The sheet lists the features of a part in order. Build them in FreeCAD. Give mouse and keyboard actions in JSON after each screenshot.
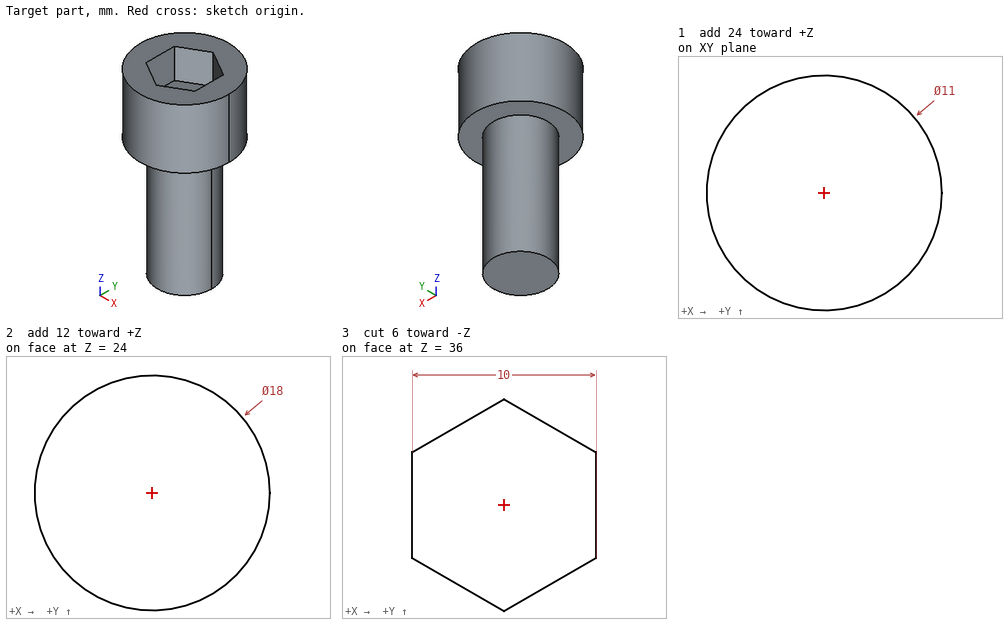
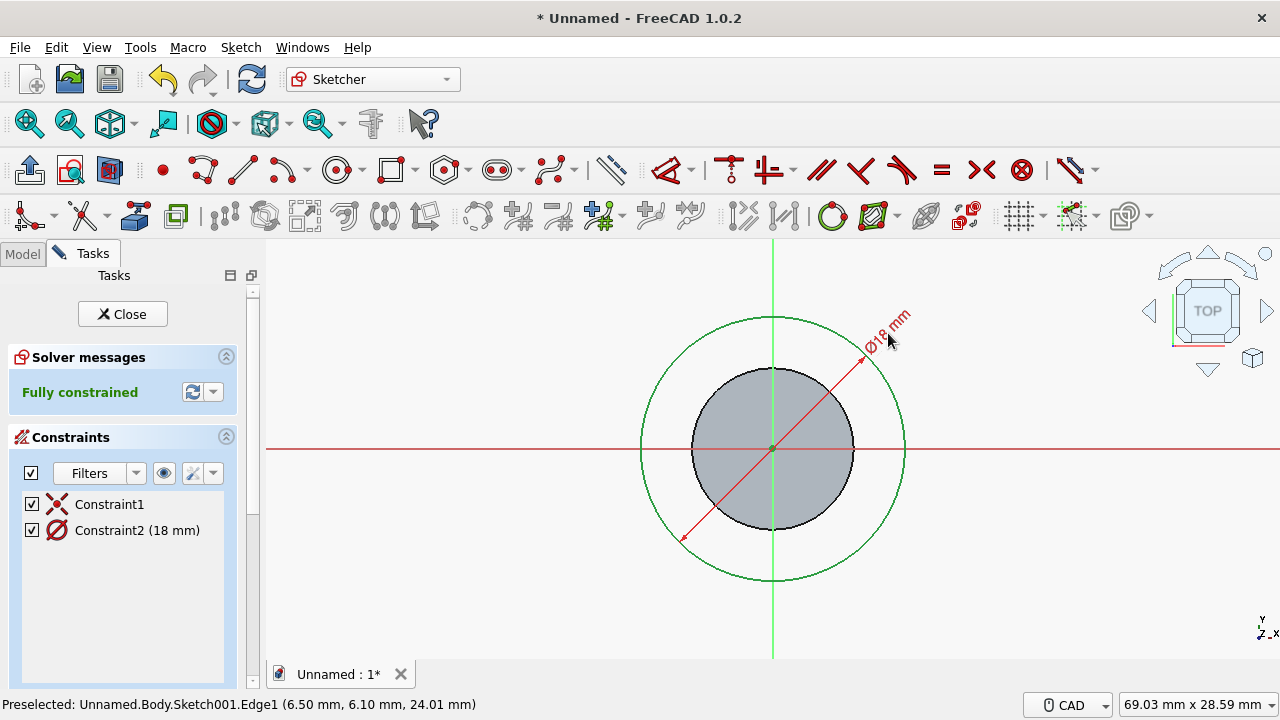
{"action": "left_click", "coordinate": [123, 314]}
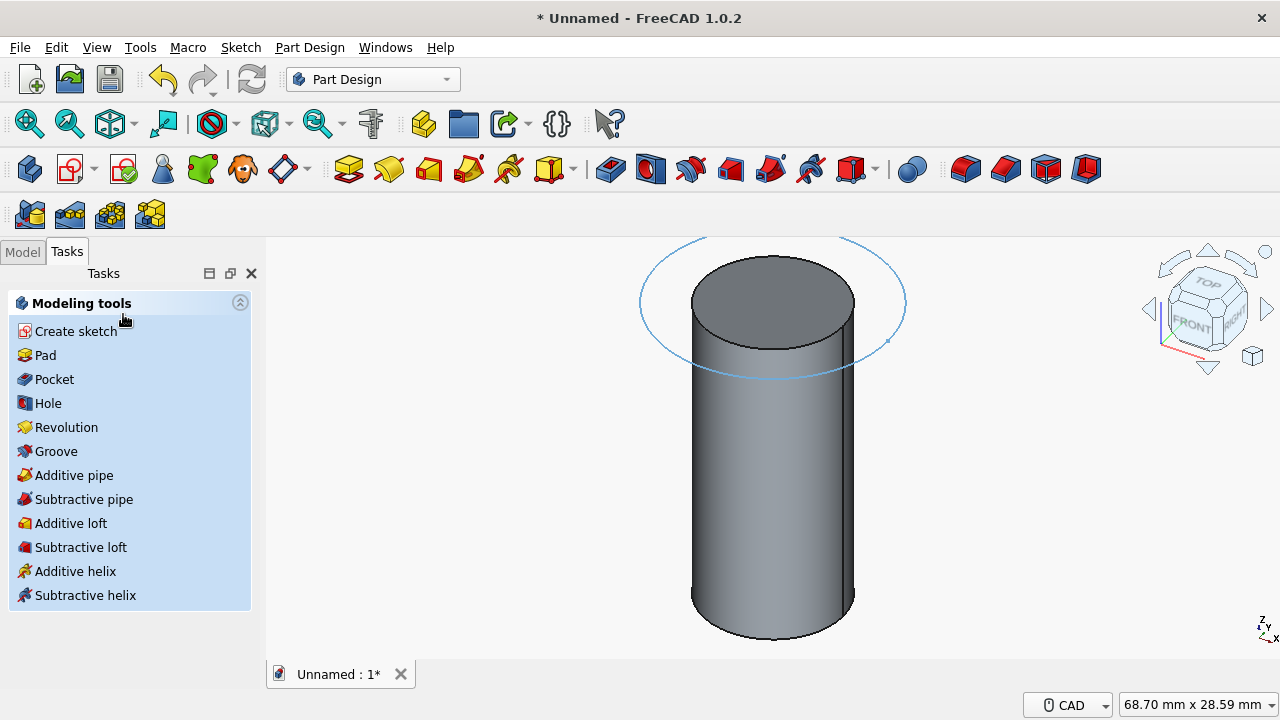
{"action": "left_click", "coordinate": [350, 170]}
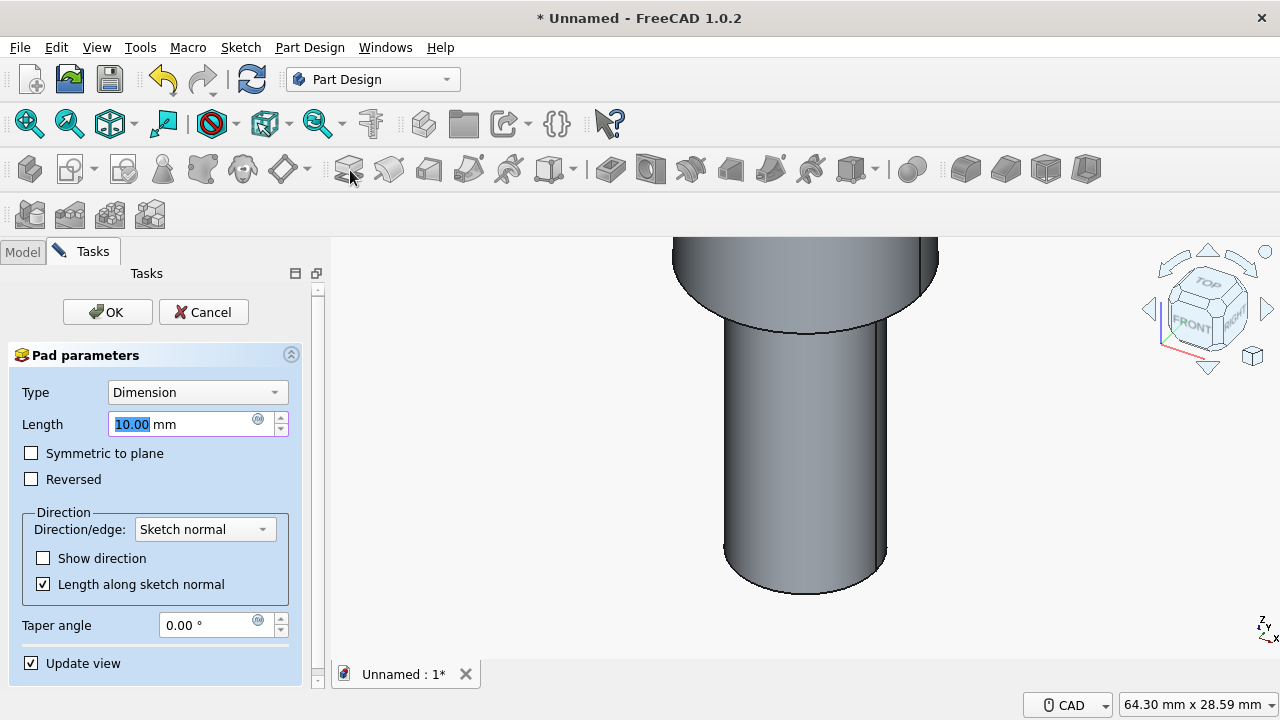
{"action": "type", "text": "12"}
{"action": "key", "text": "Tab"}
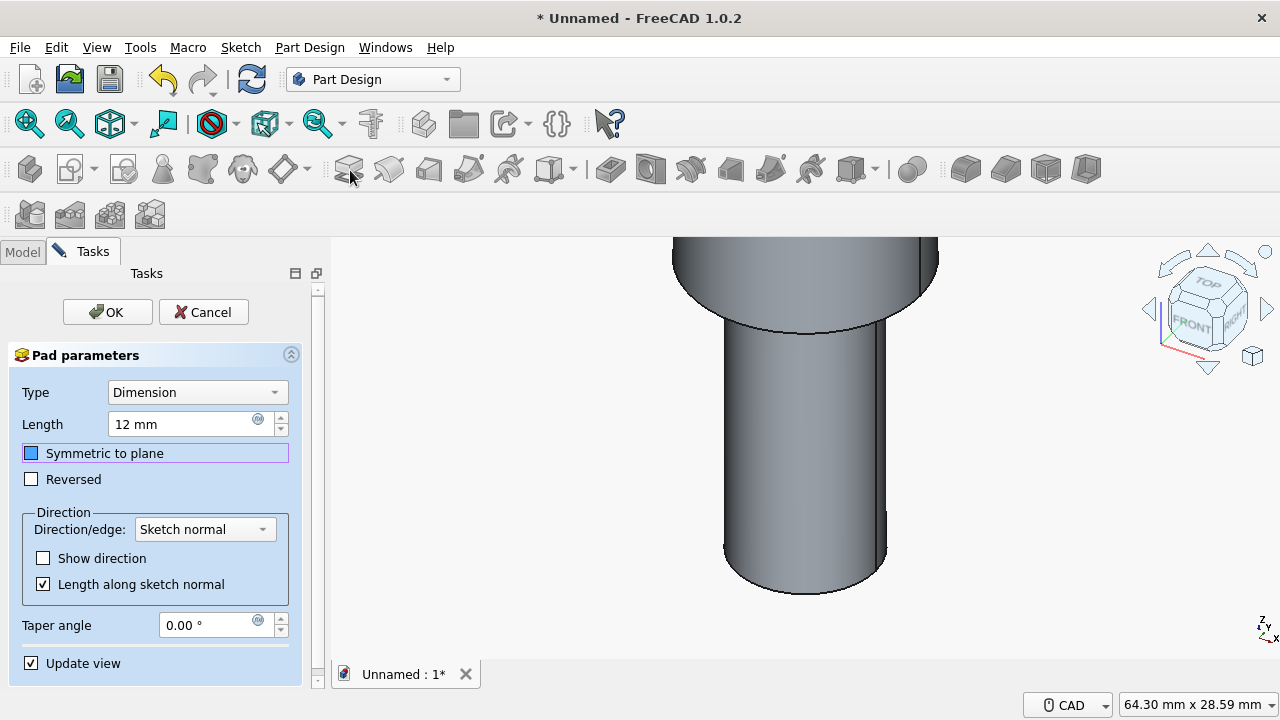
{"action": "left_click", "coordinate": [108, 312]}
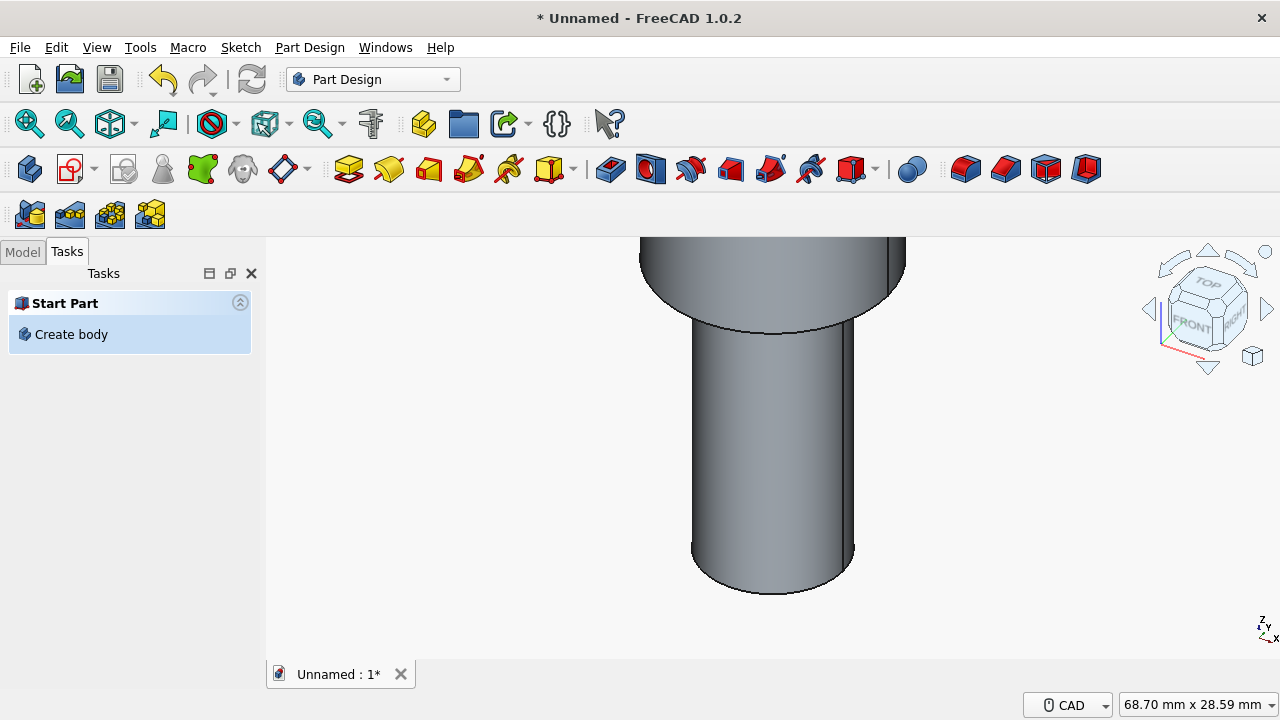
{"action": "left_click", "coordinate": [30, 124]}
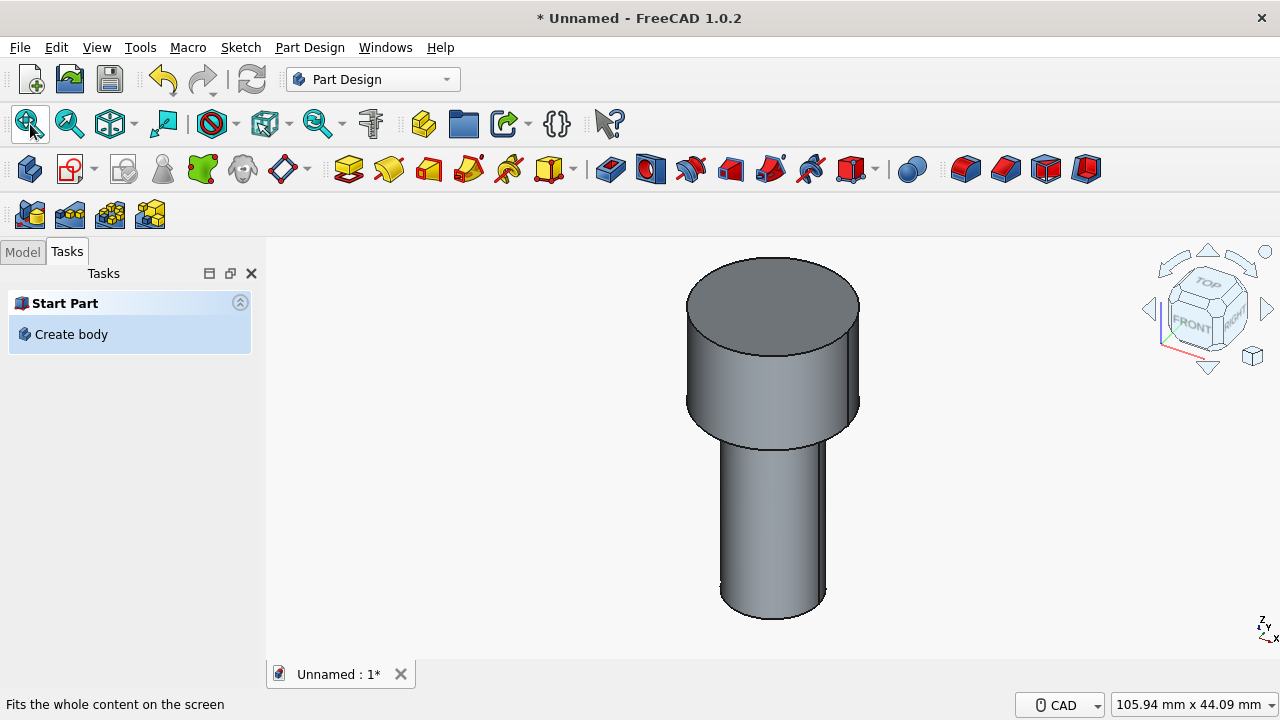
{"action": "left_click", "coordinate": [773, 306]}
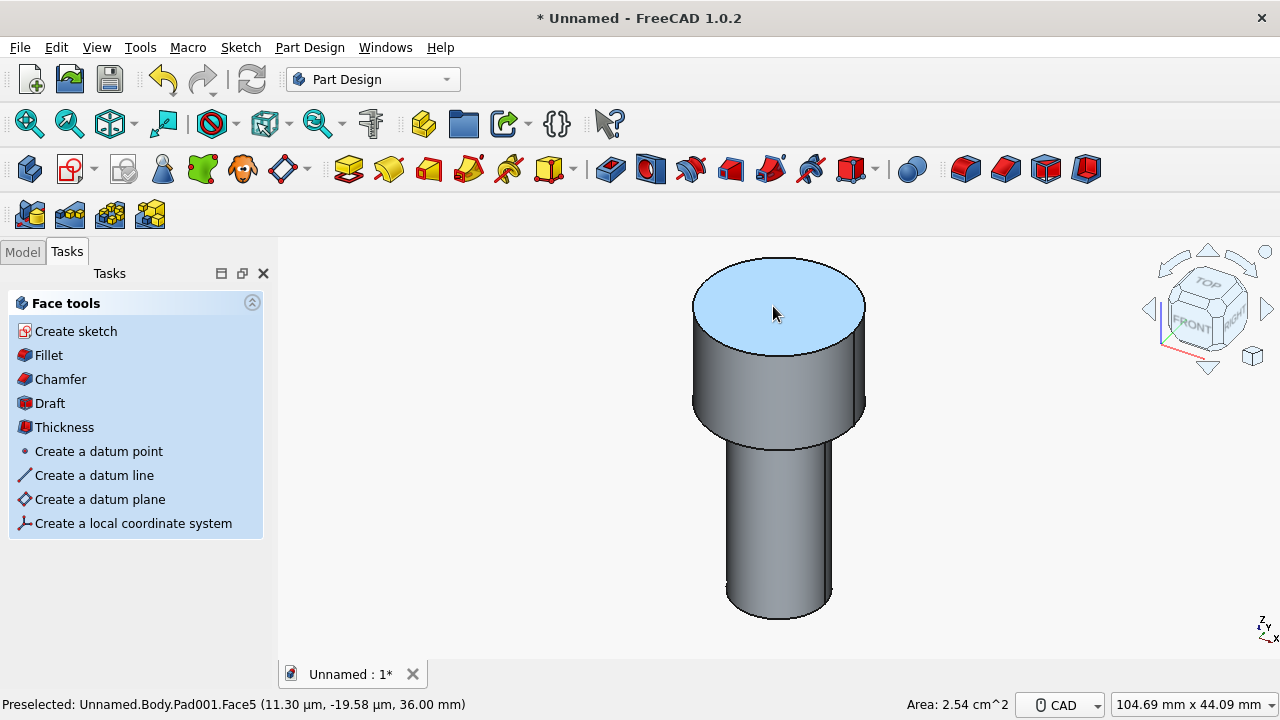
{"action": "left_click", "coordinate": [70, 170]}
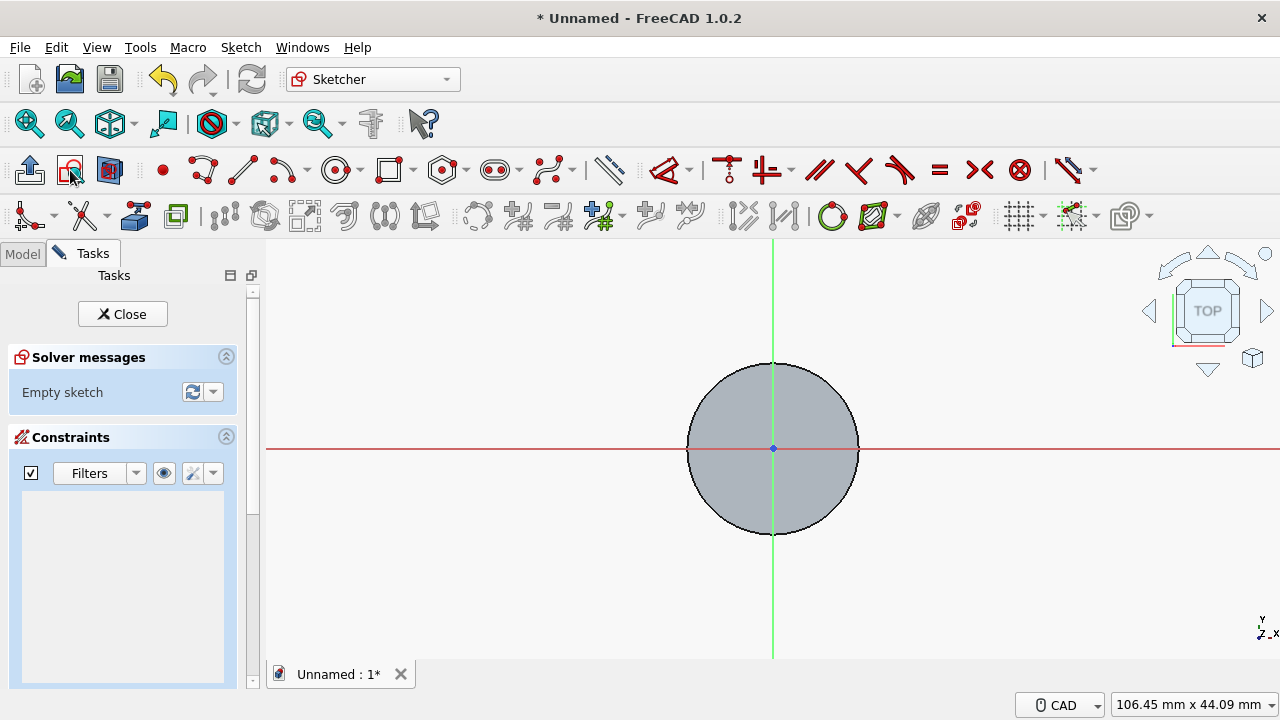
{"action": "scroll", "coordinate": [829, 449], "scroll_direction": "up", "scroll_amount": 4}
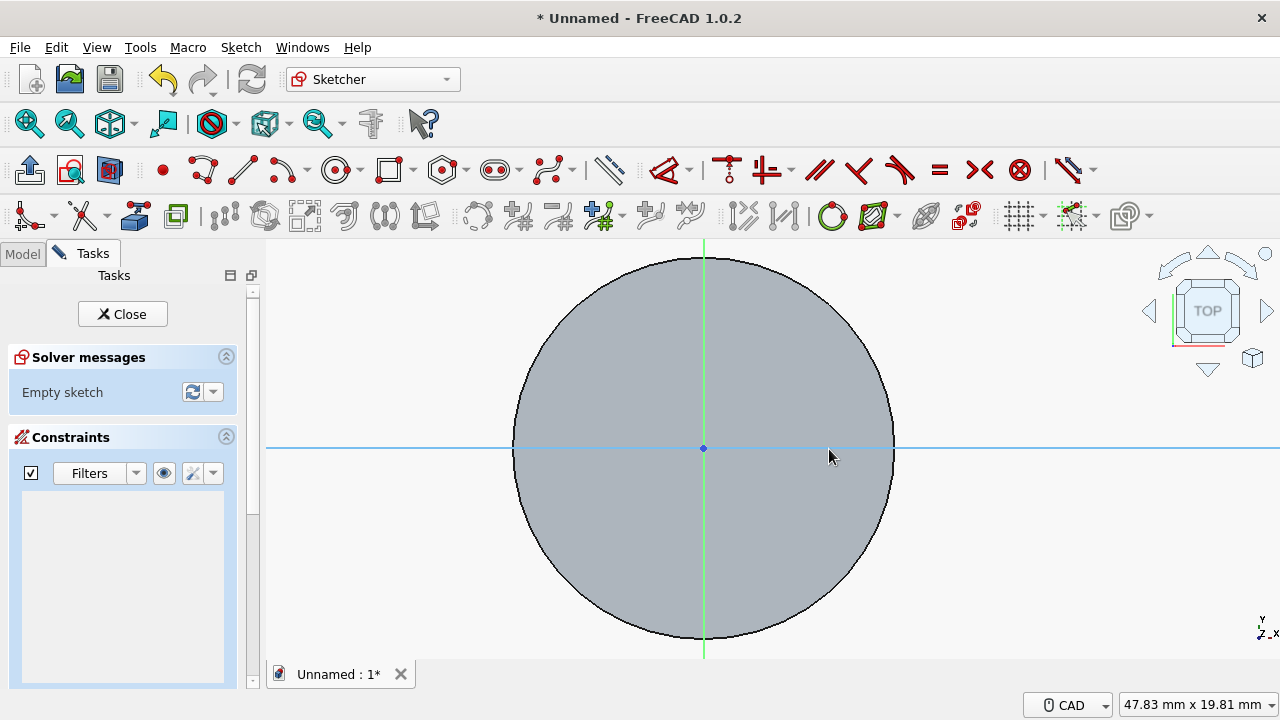
{"action": "left_click", "coordinate": [442, 170]}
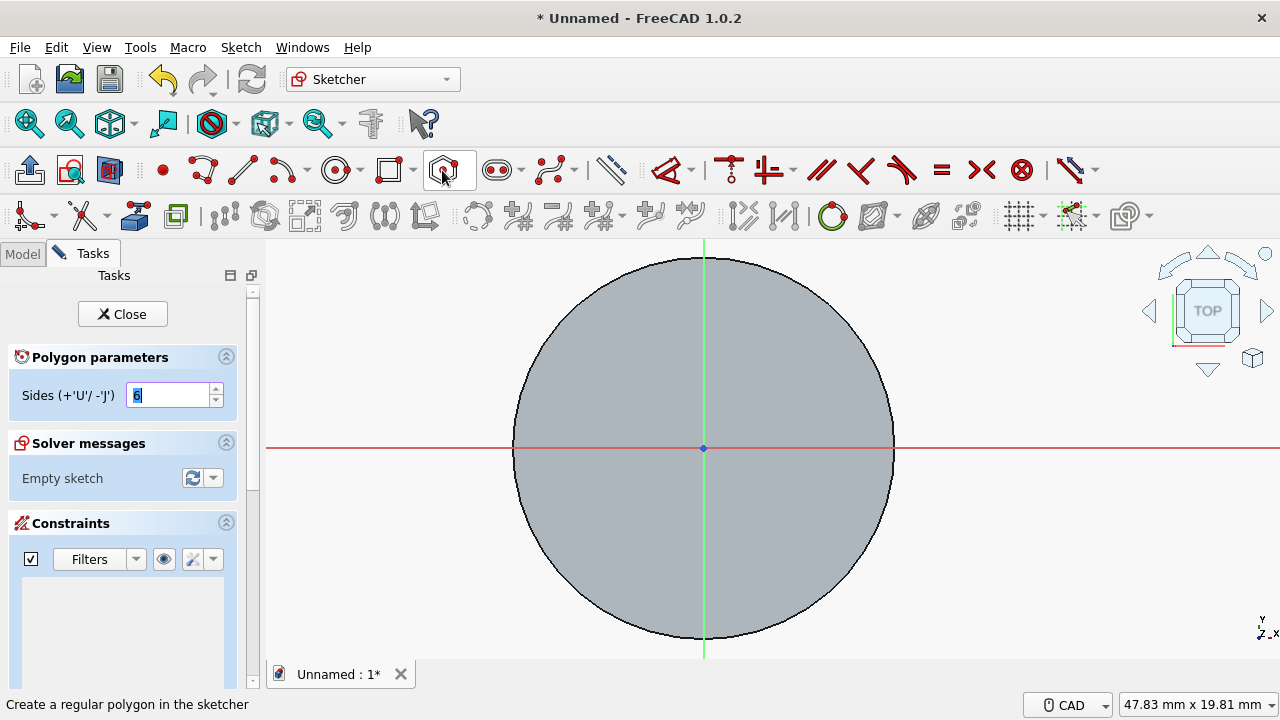
{"action": "left_click", "coordinate": [704, 448]}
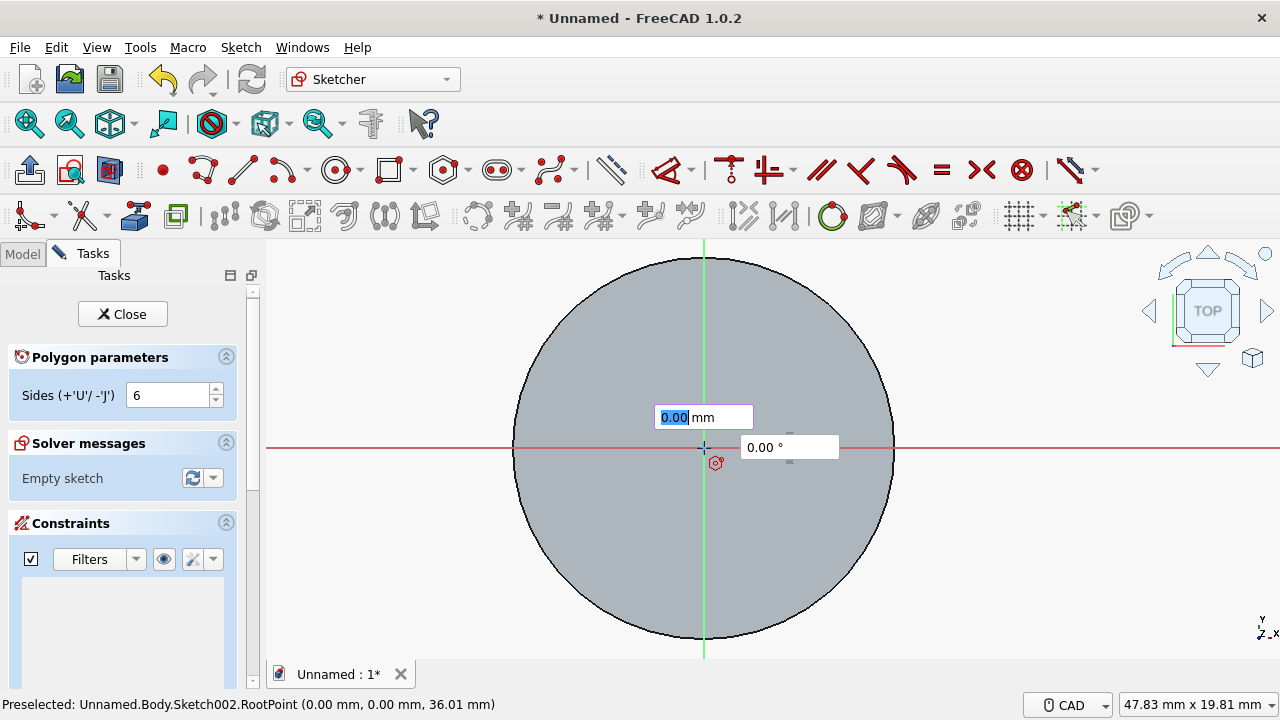
{"action": "left_click", "coordinate": [704, 326]}
{"action": "right_click", "coordinate": [704, 326]}